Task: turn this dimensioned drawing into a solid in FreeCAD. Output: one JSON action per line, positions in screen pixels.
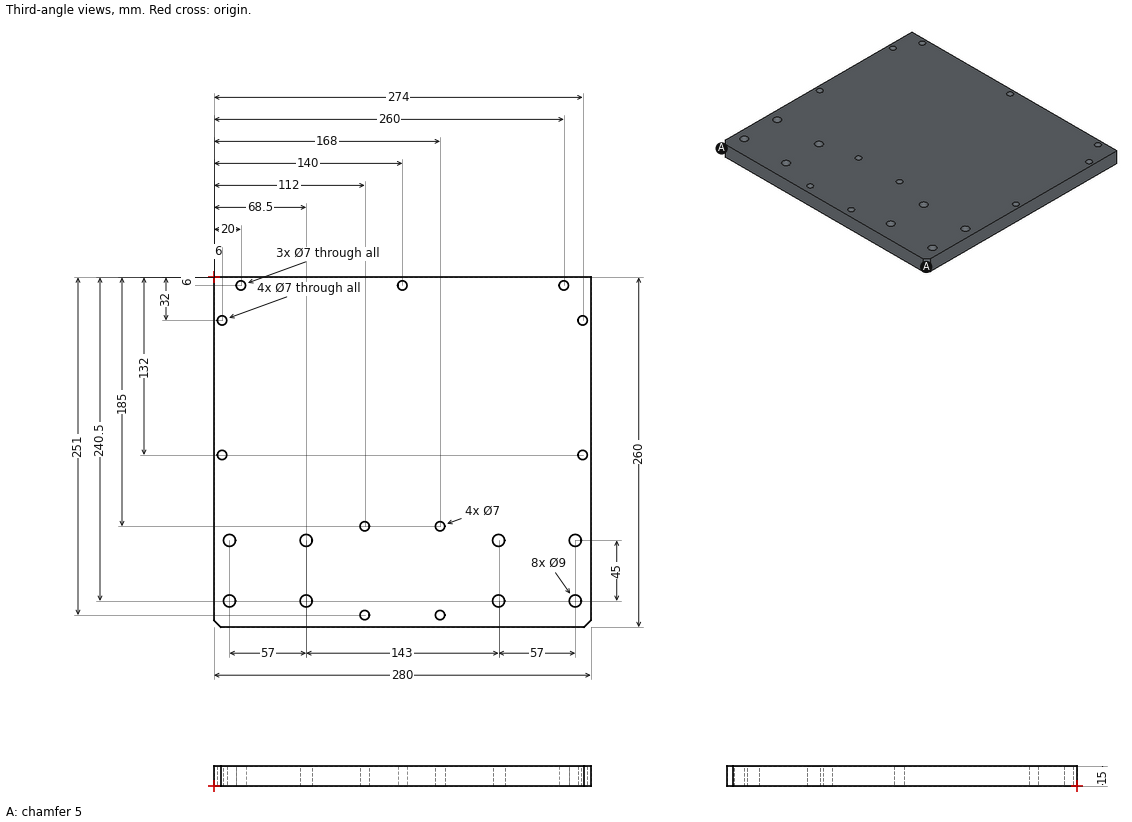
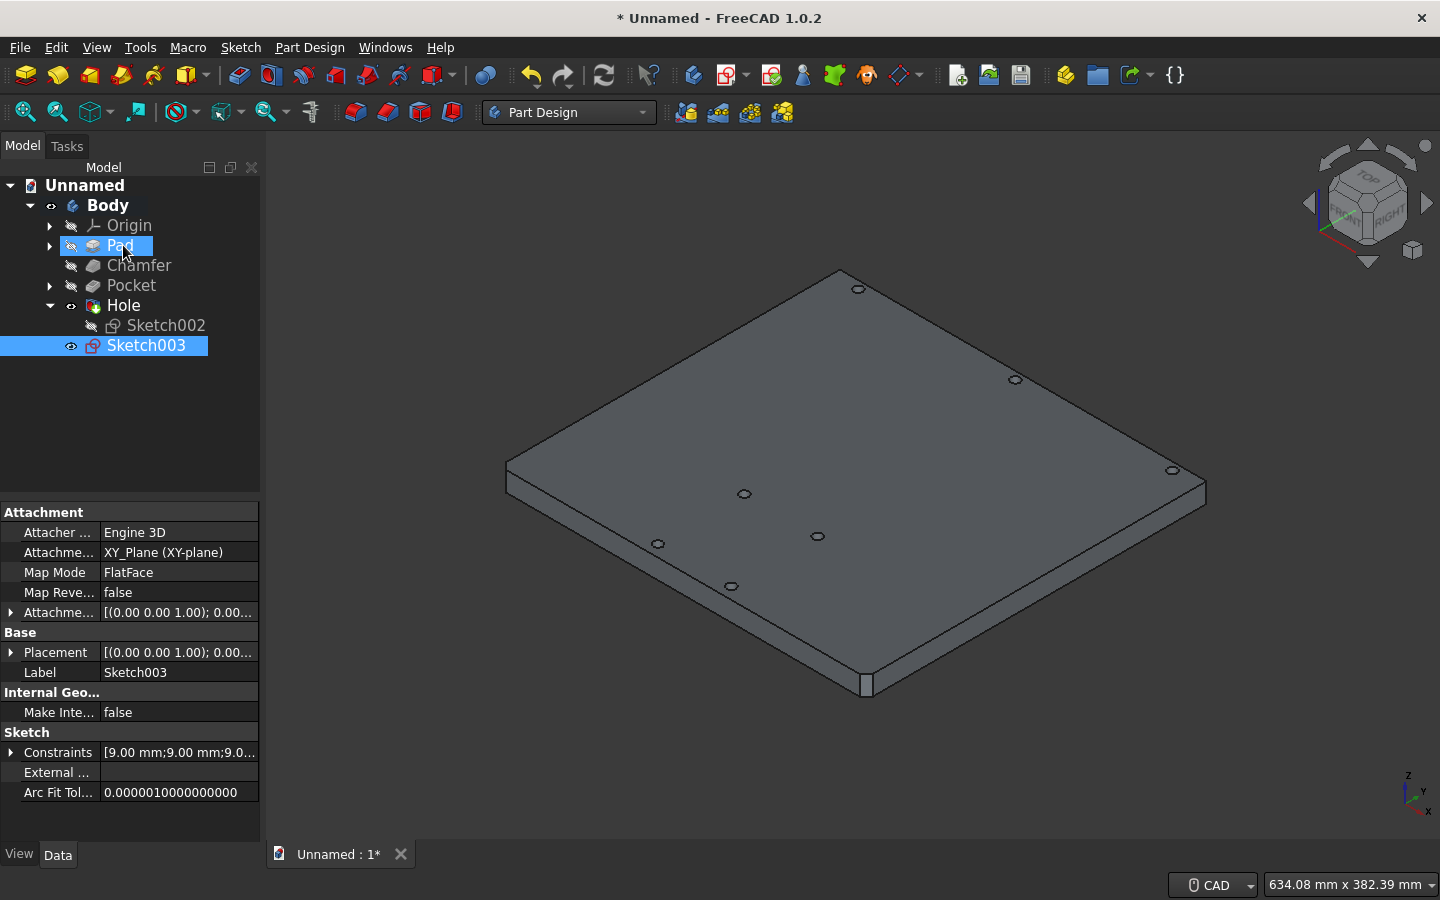
{"action": "left_click", "coordinate": [240, 76]}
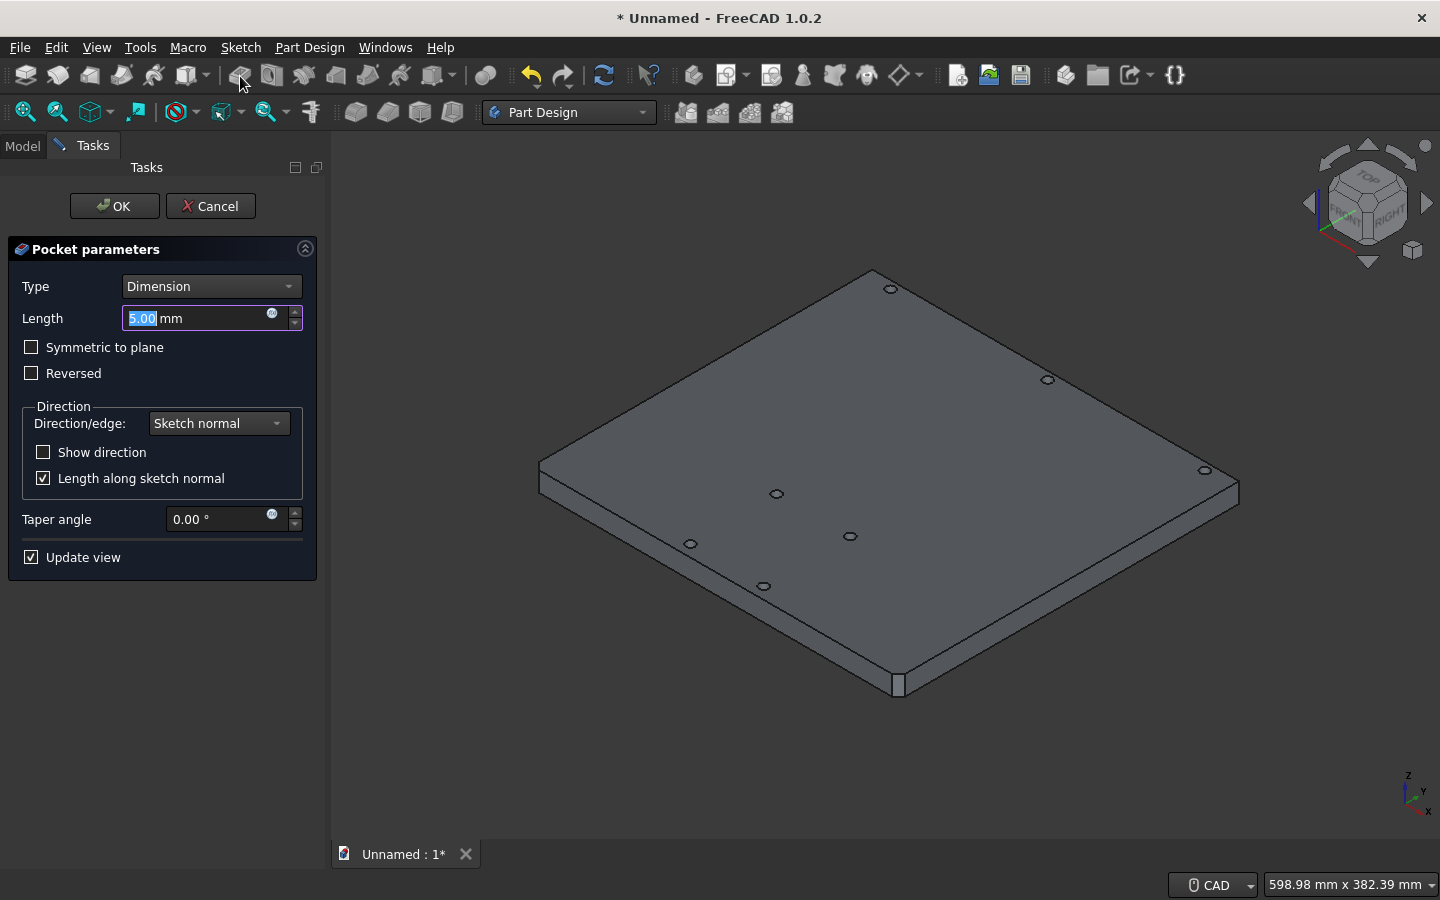
{"action": "left_click", "coordinate": [212, 286]}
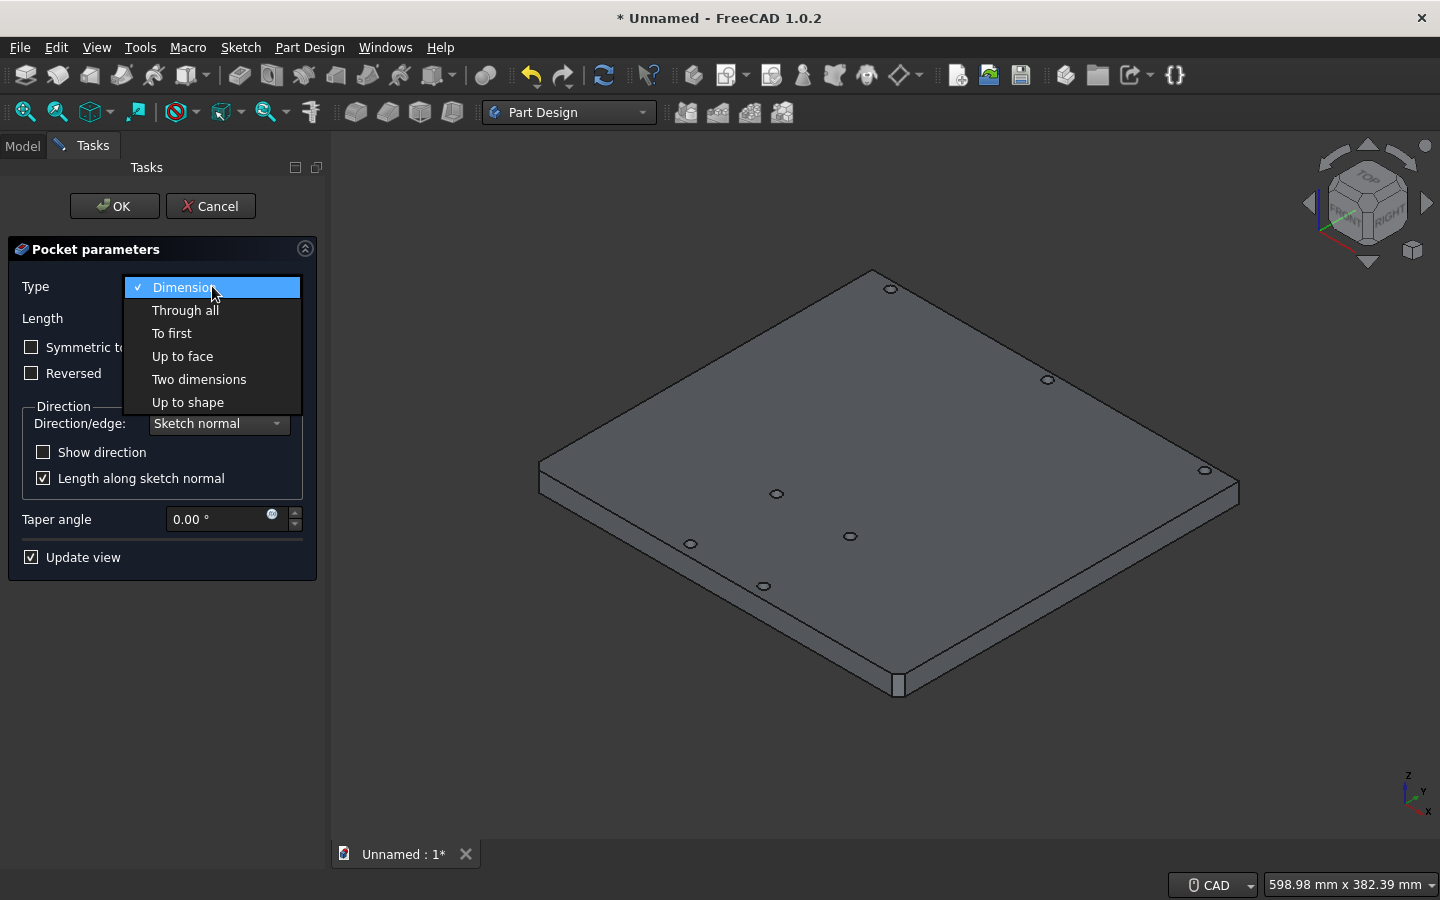
{"action": "left_click", "coordinate": [212, 310]}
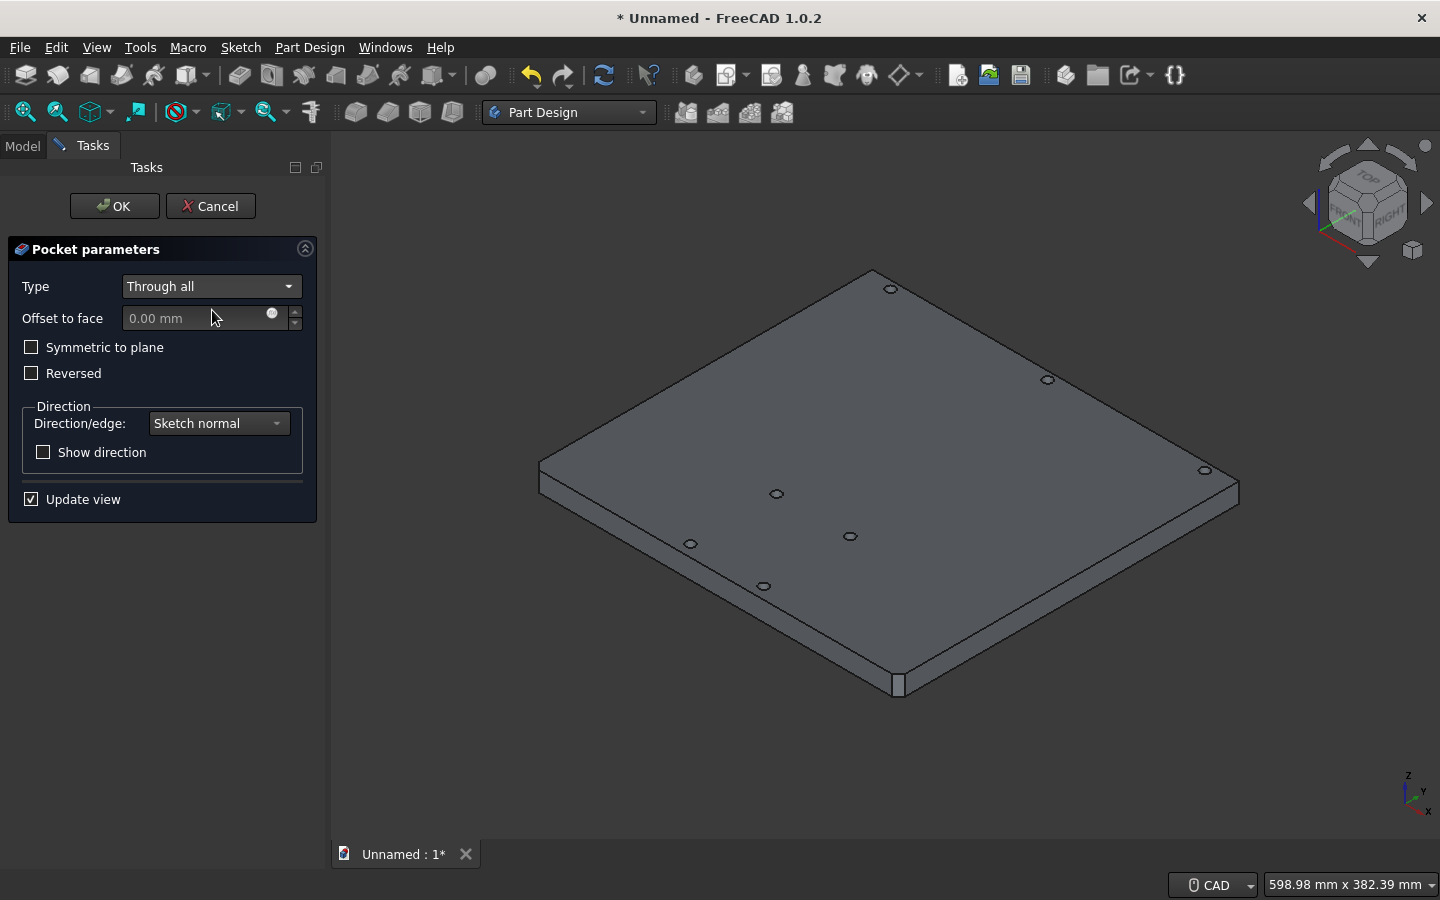
{"action": "left_click", "coordinate": [30, 373]}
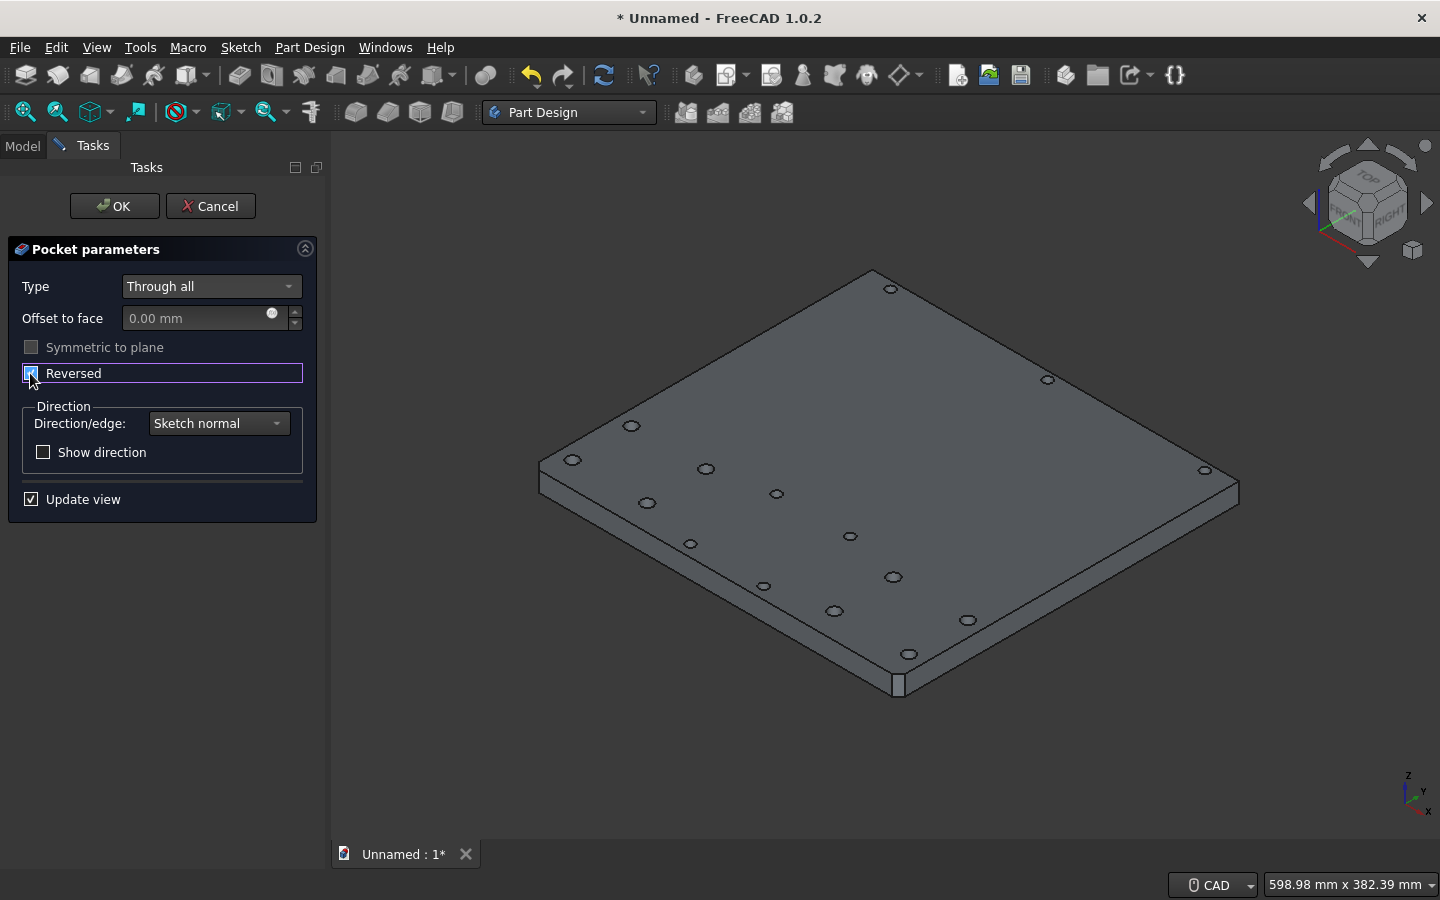
{"action": "left_click", "coordinate": [115, 206]}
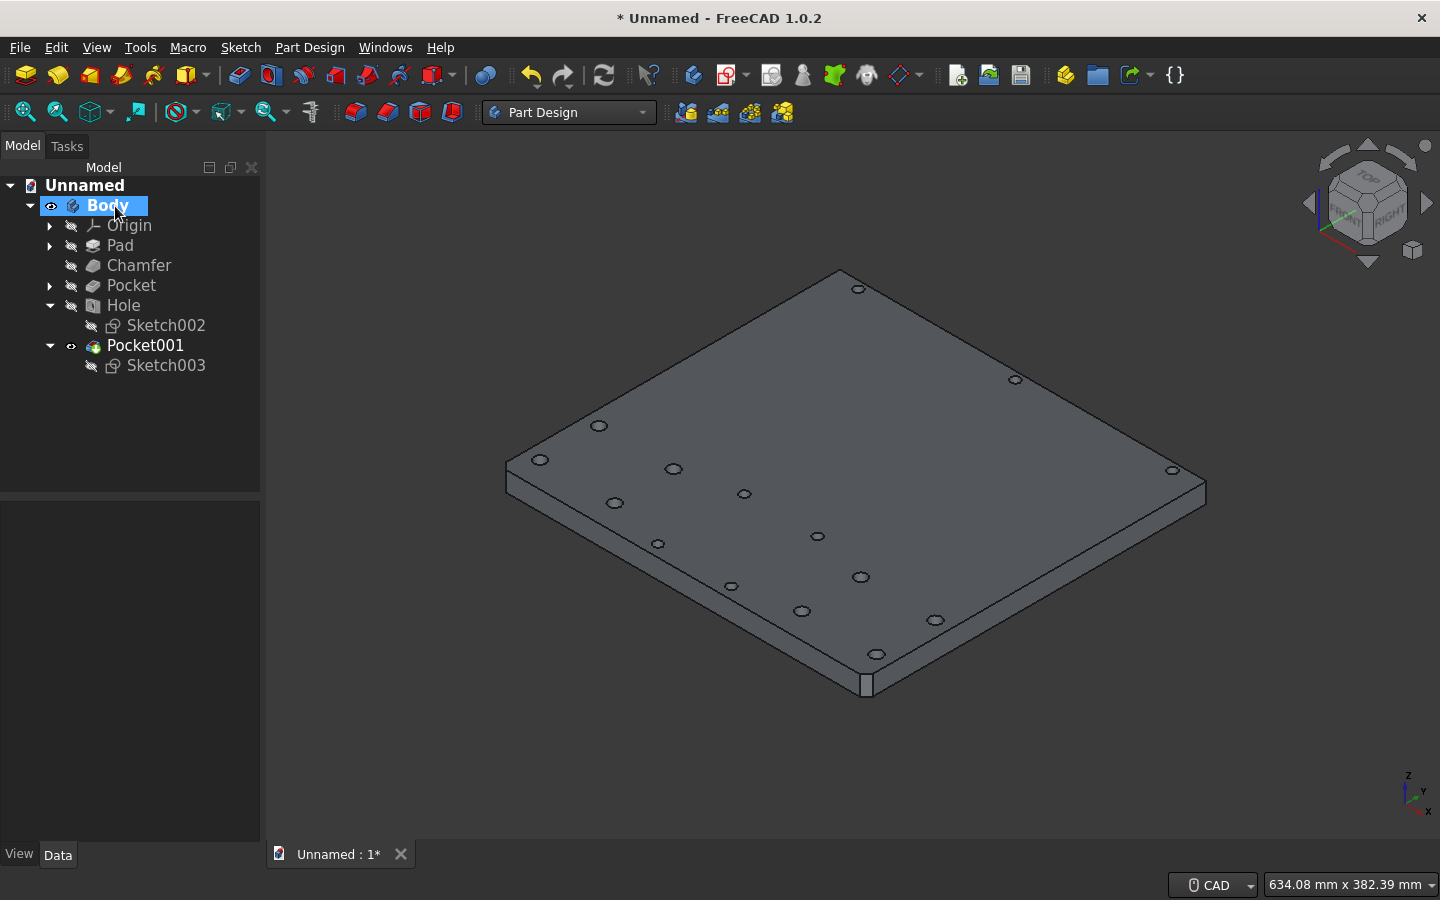
{"action": "left_click", "coordinate": [954, 475]}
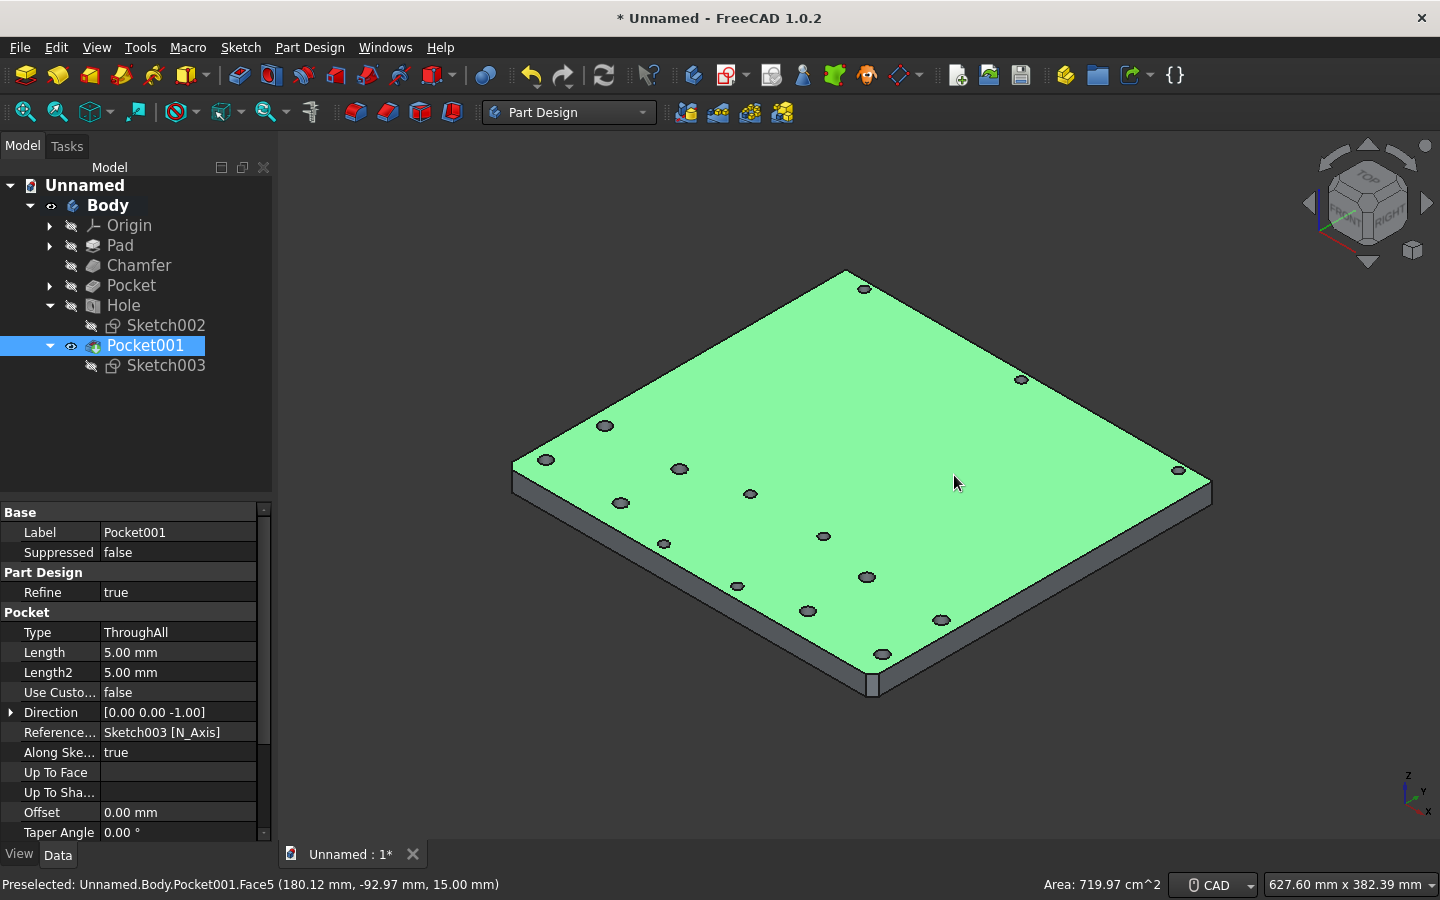
{"action": "left_click", "coordinate": [726, 76]}